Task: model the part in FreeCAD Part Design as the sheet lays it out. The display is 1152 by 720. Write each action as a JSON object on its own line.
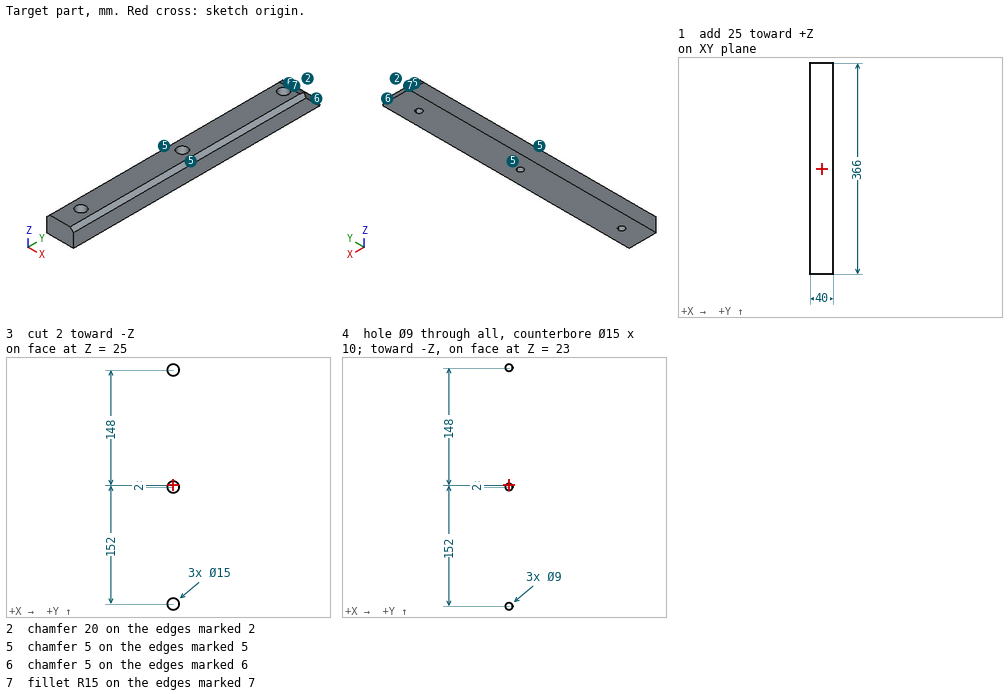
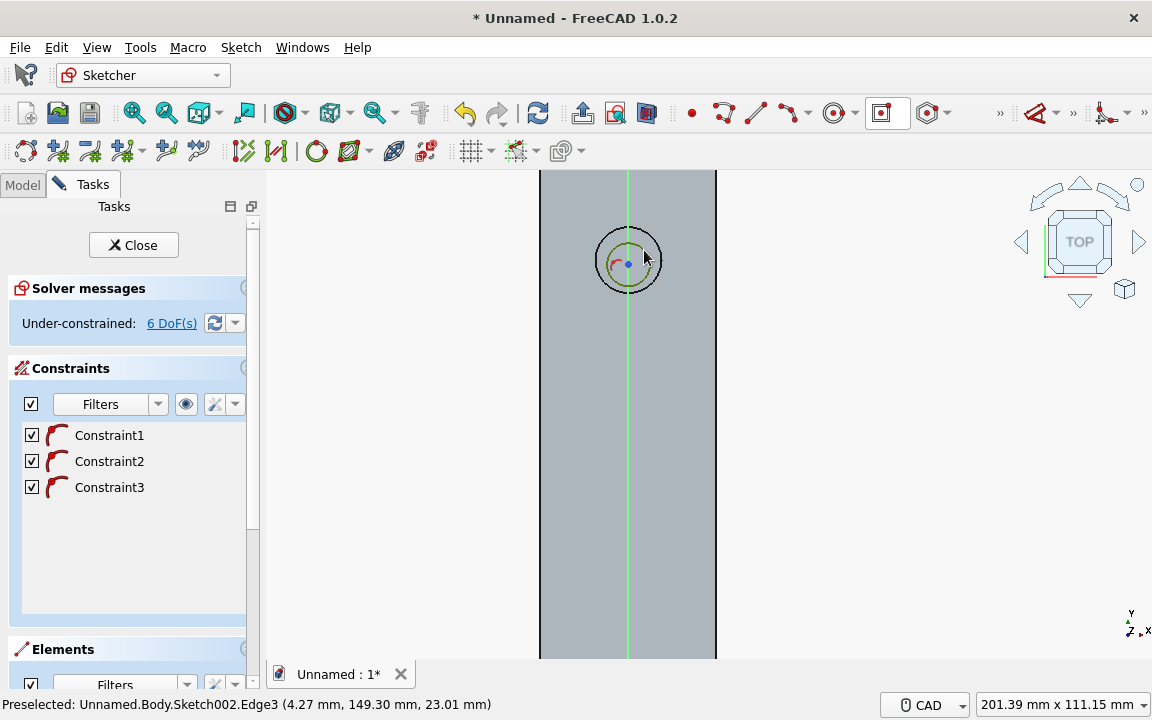
{"action": "key", "text": "e"}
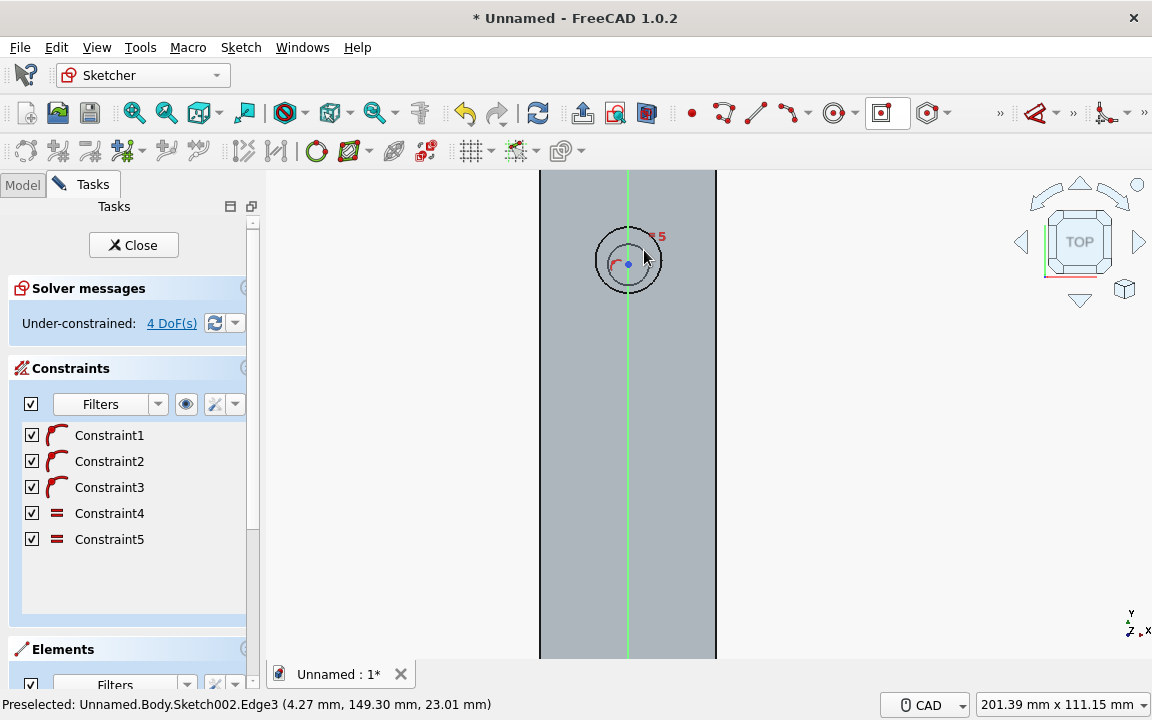
{"action": "left_click", "coordinate": [1036, 114]}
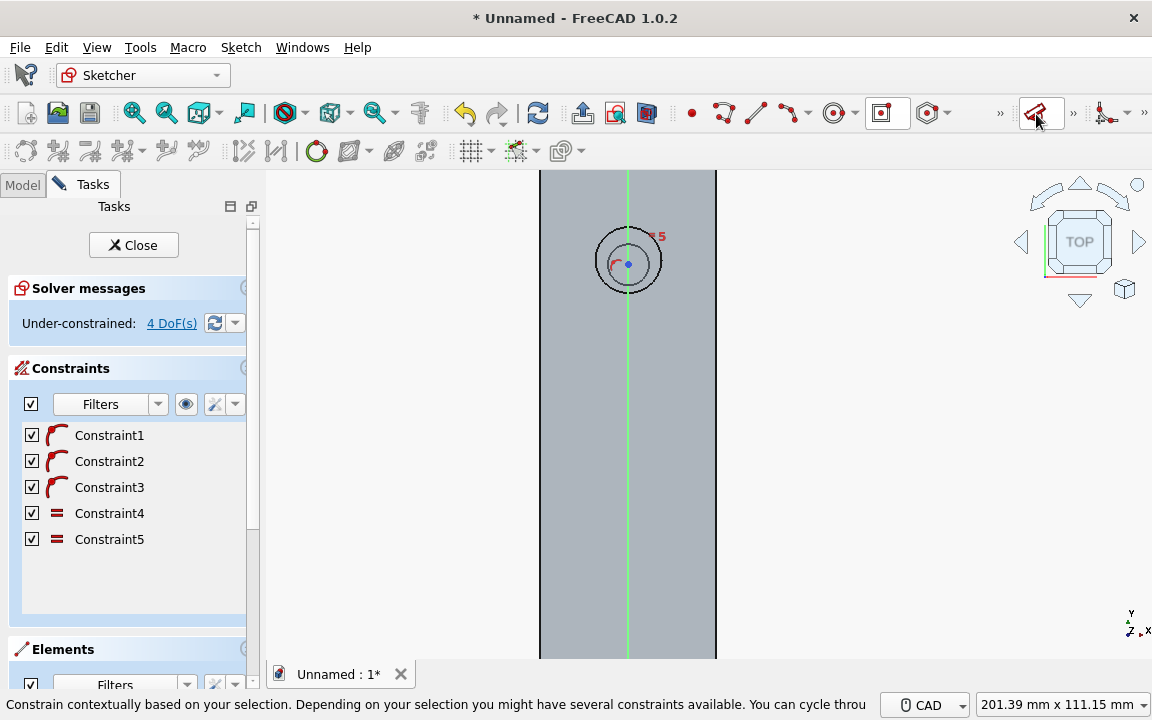
{"action": "scroll", "coordinate": [644, 249], "scroll_direction": "down", "scroll_amount": 7}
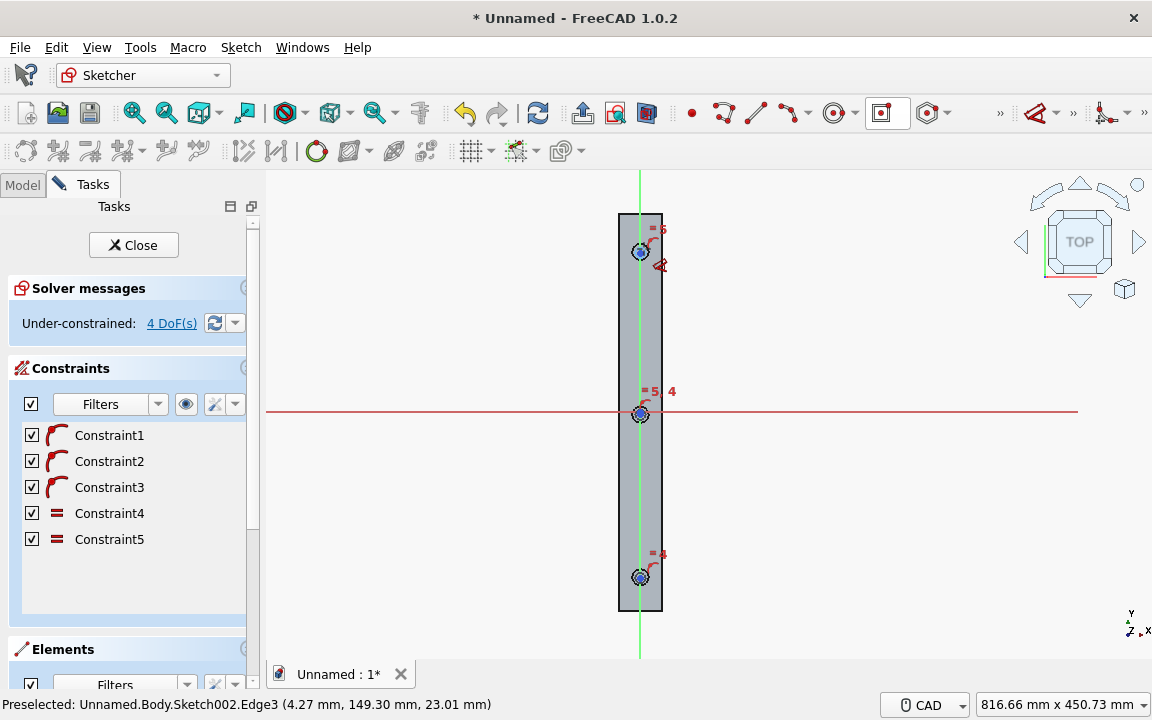
{"action": "scroll", "coordinate": [644, 575], "scroll_direction": "up", "scroll_amount": 8}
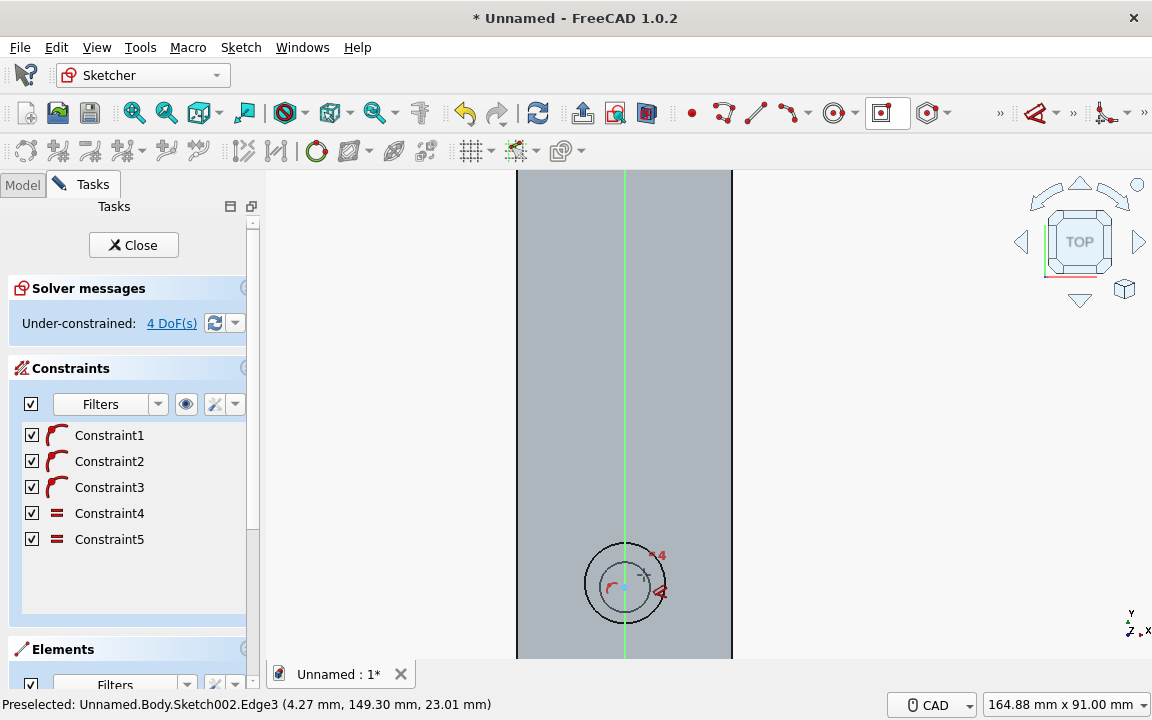
{"action": "left_click", "coordinate": [643, 570]}
{"action": "left_click", "coordinate": [666, 548]}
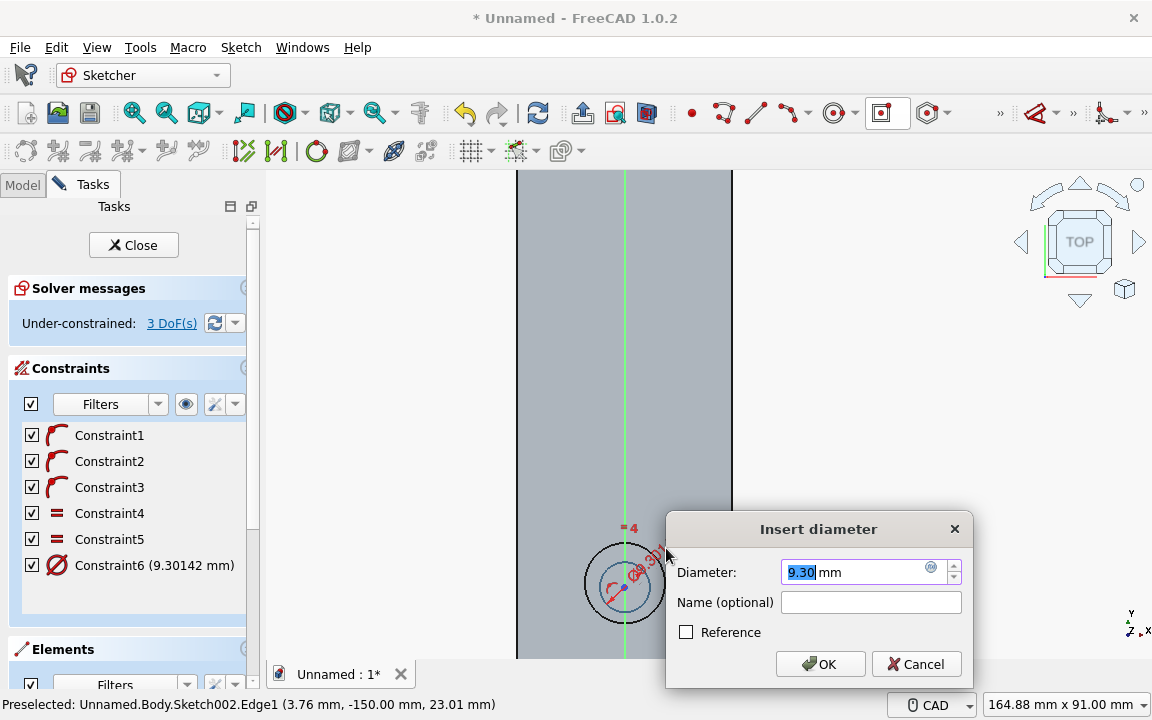
{"action": "type", "text": "9"}
{"action": "key", "text": "Return"}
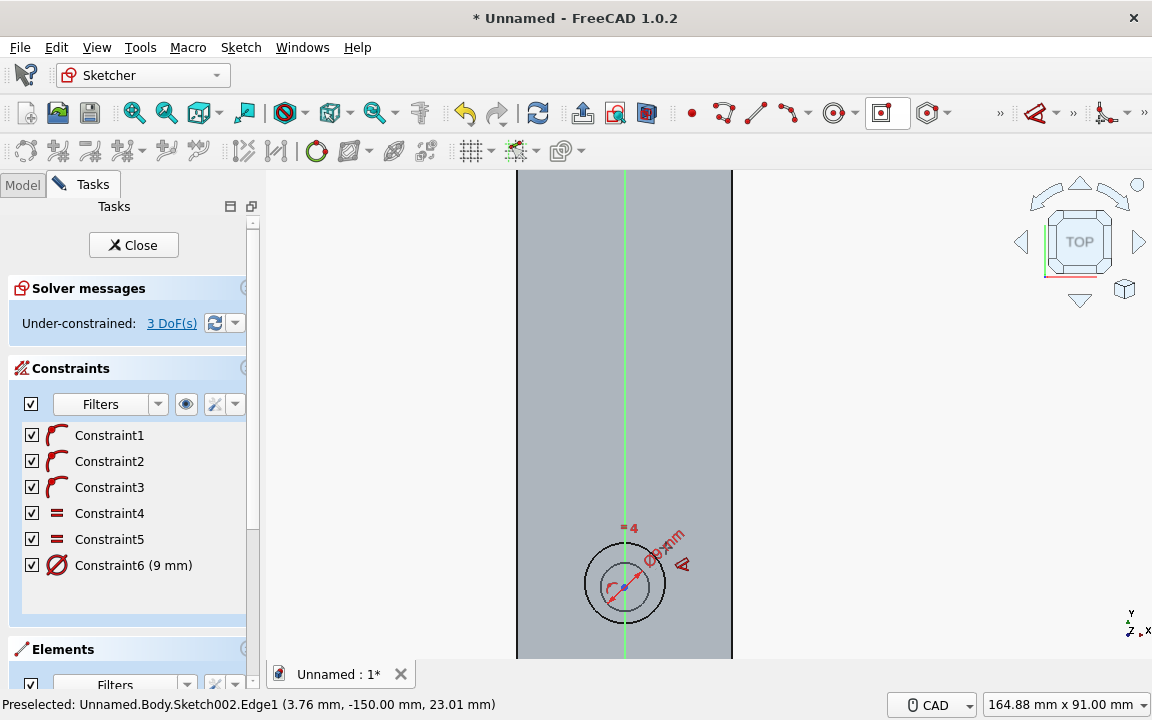
{"action": "scroll", "coordinate": [644, 576], "scroll_direction": "down", "scroll_amount": 8}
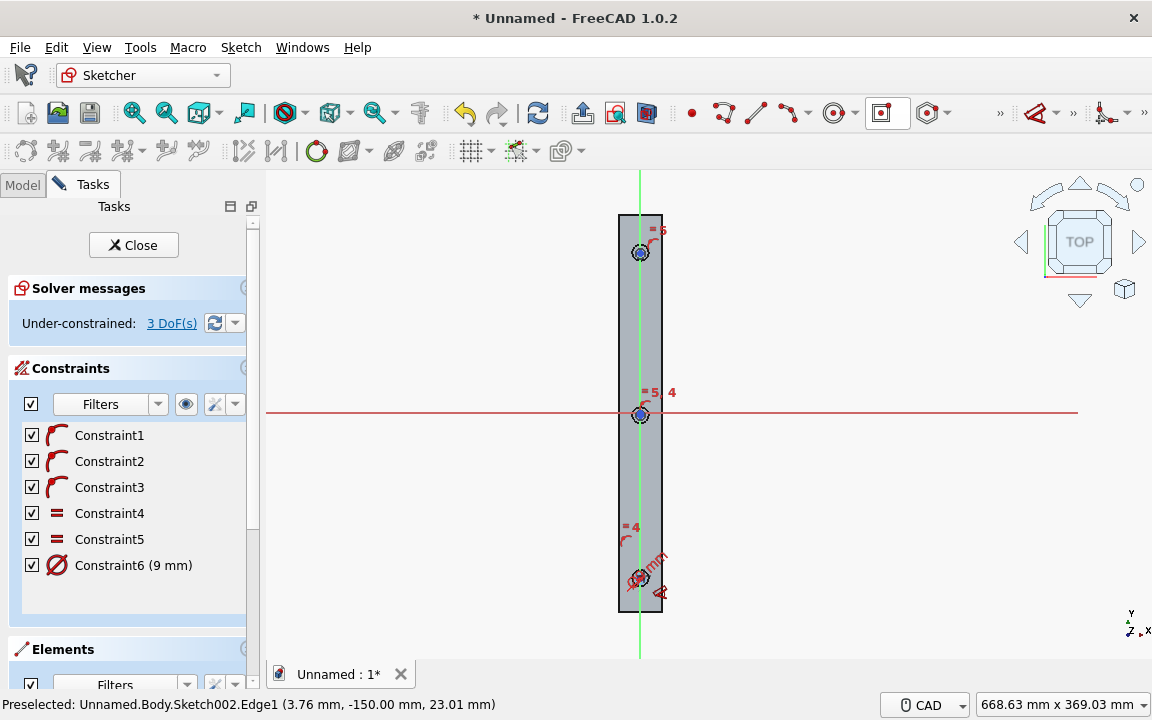
{"action": "scroll", "coordinate": [640, 416], "scroll_direction": "up", "scroll_amount": 15}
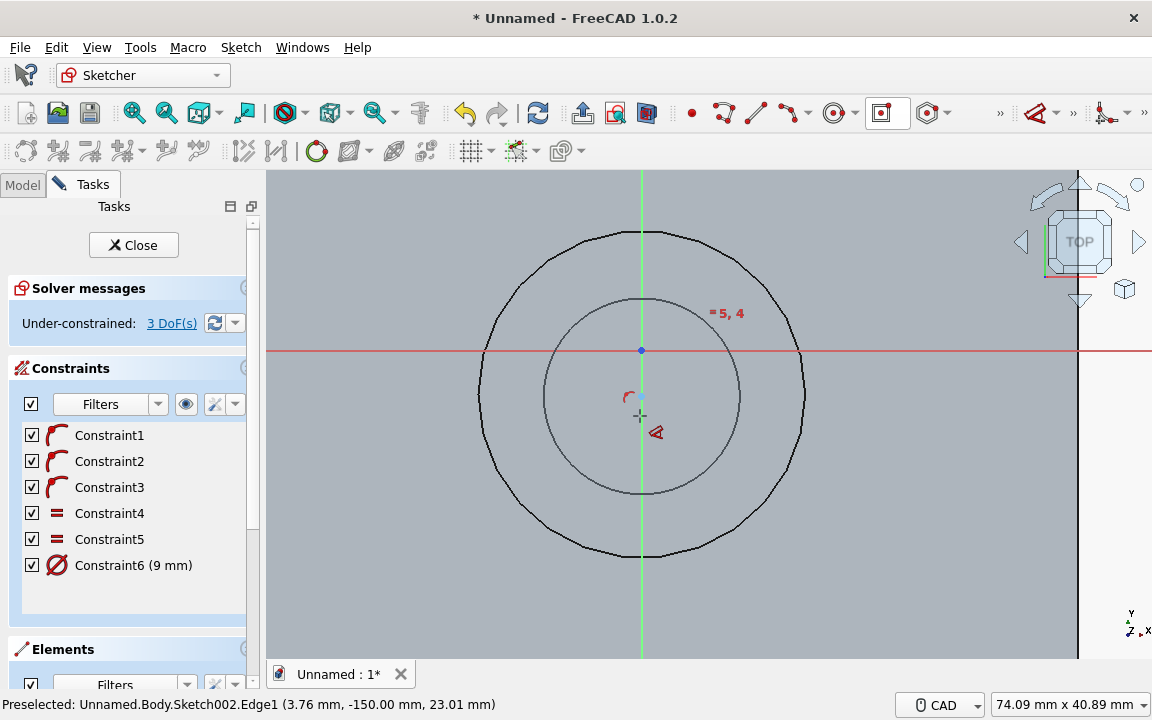
{"action": "left_click", "coordinate": [642, 396]}
{"action": "left_click", "coordinate": [676, 374]}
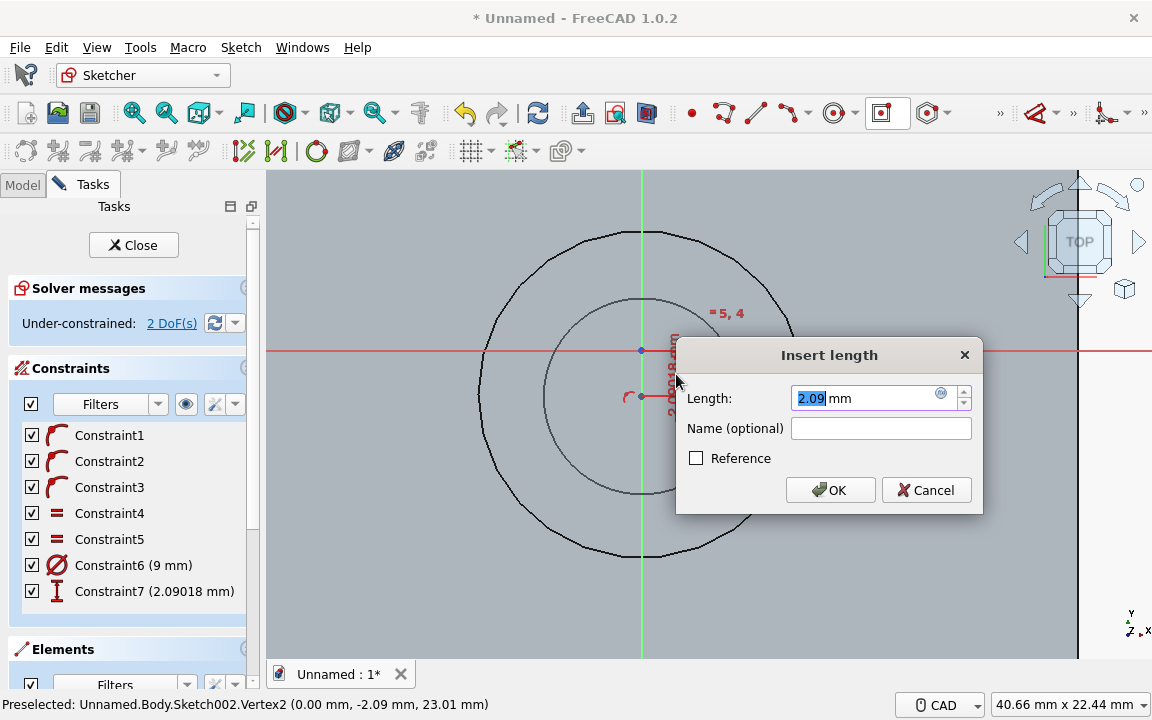
{"action": "type", "text": "2"}
{"action": "key", "text": "Return"}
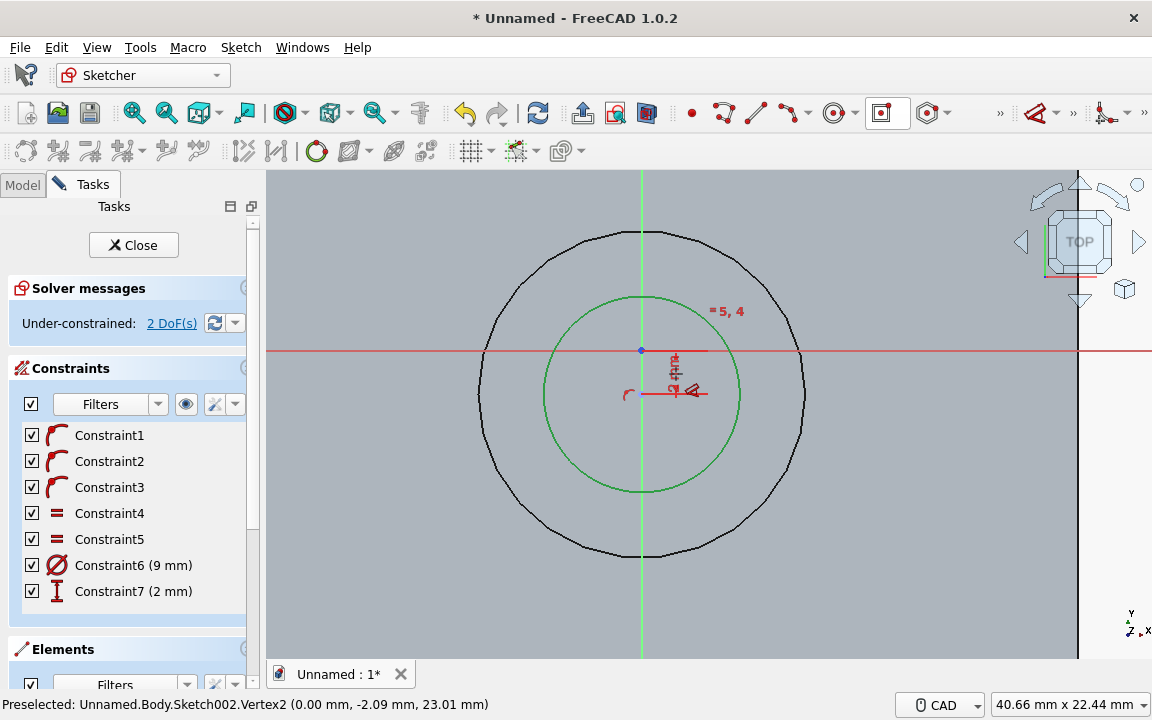
{"action": "scroll", "coordinate": [640, 416], "scroll_direction": "down", "scroll_amount": 15}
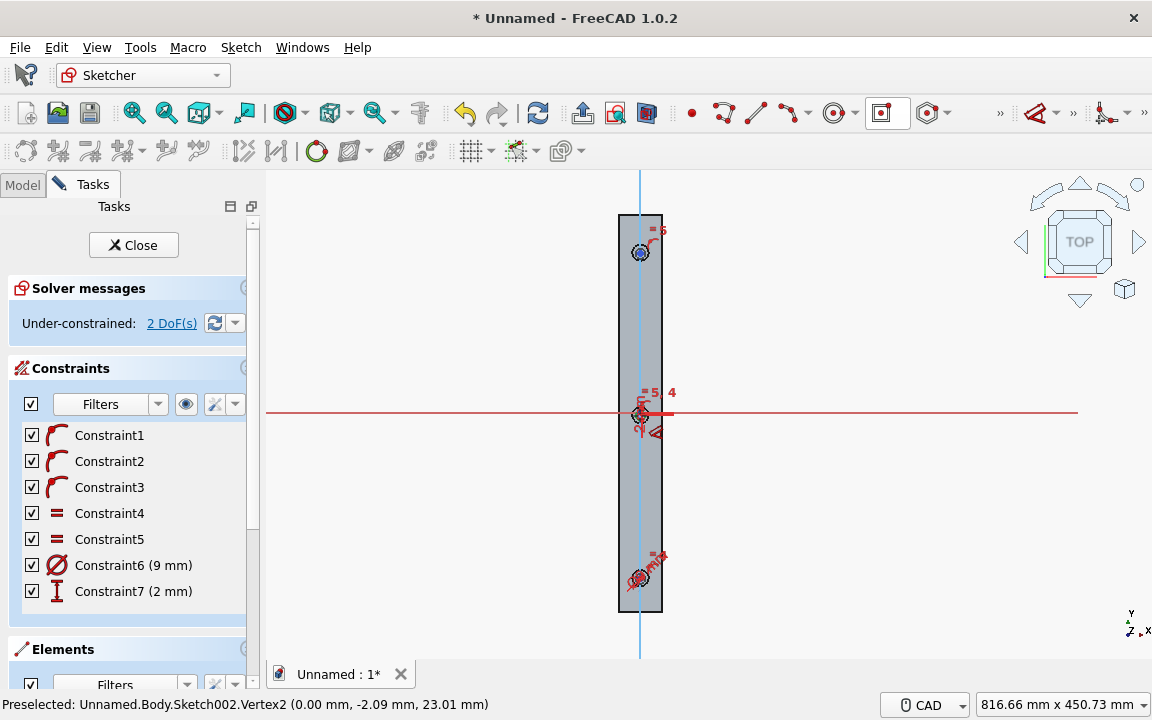
{"action": "left_click", "coordinate": [640, 579]}
{"action": "left_click", "coordinate": [674, 496]}